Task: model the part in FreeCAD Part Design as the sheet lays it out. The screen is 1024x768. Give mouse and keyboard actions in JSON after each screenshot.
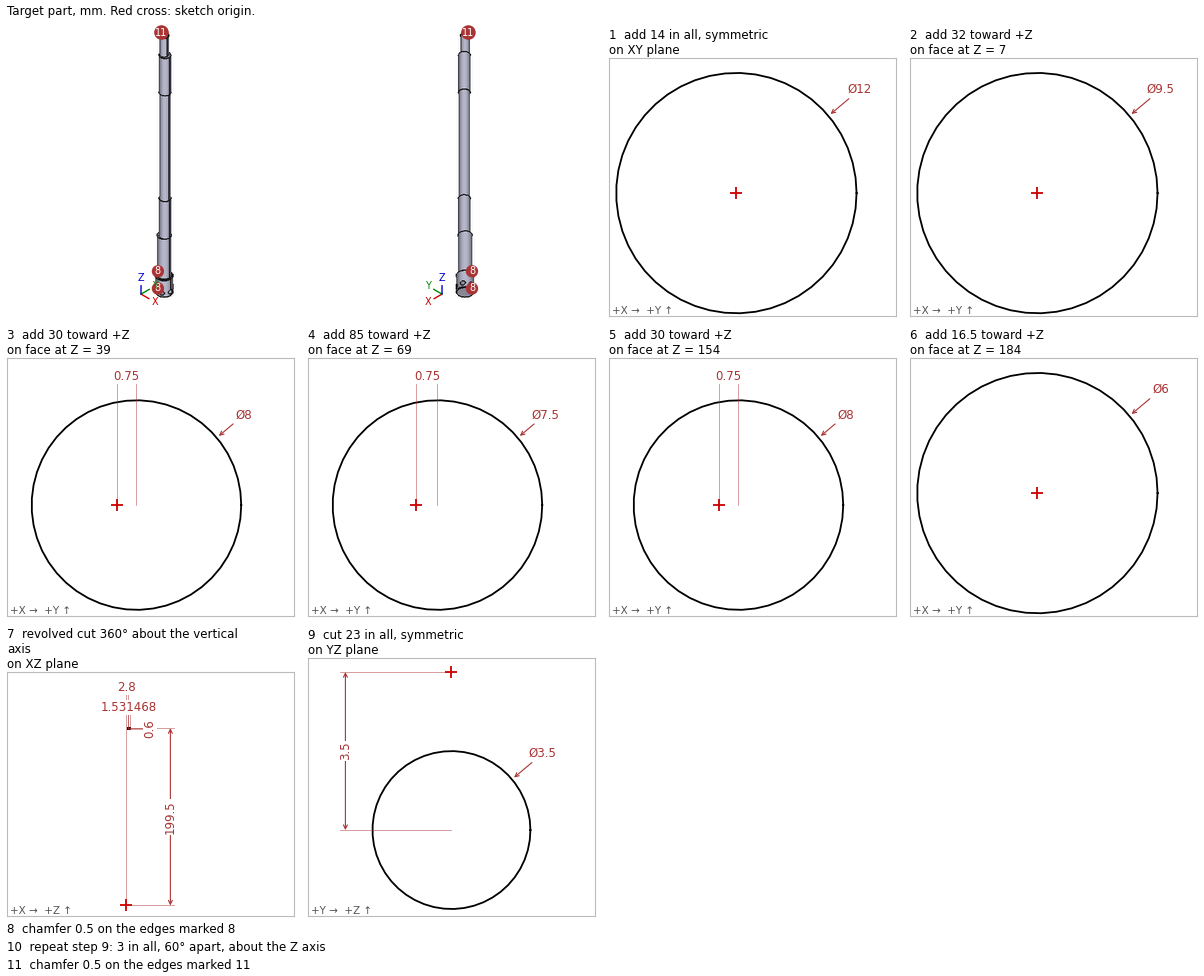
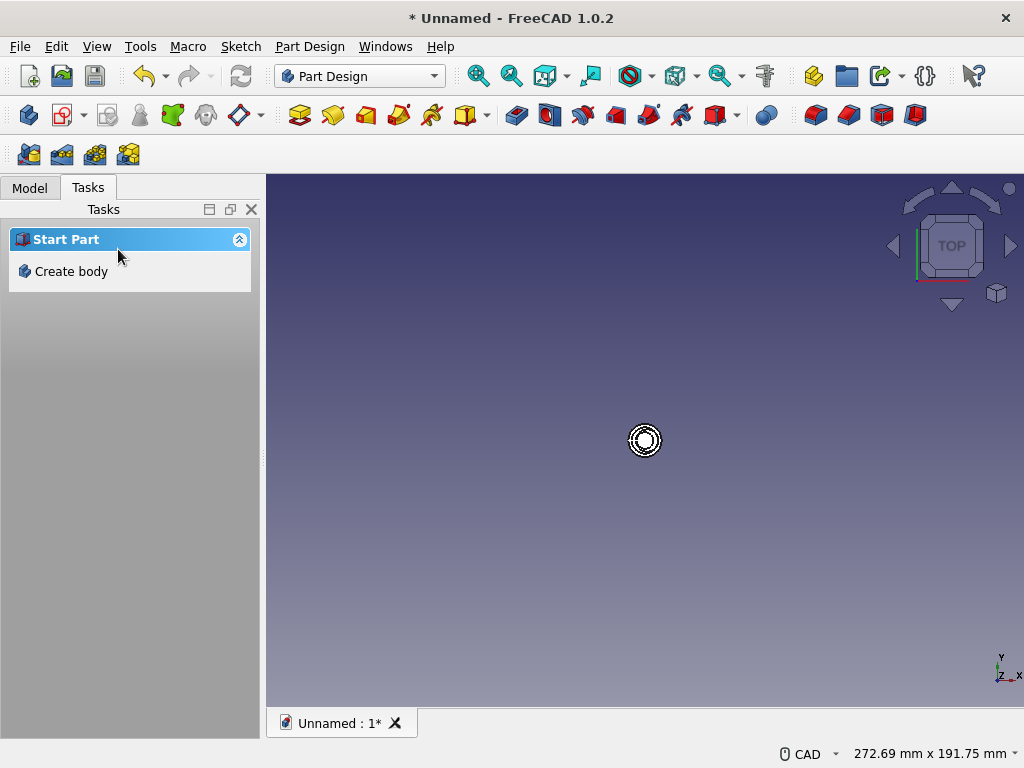
{"action": "key", "text": "v f"}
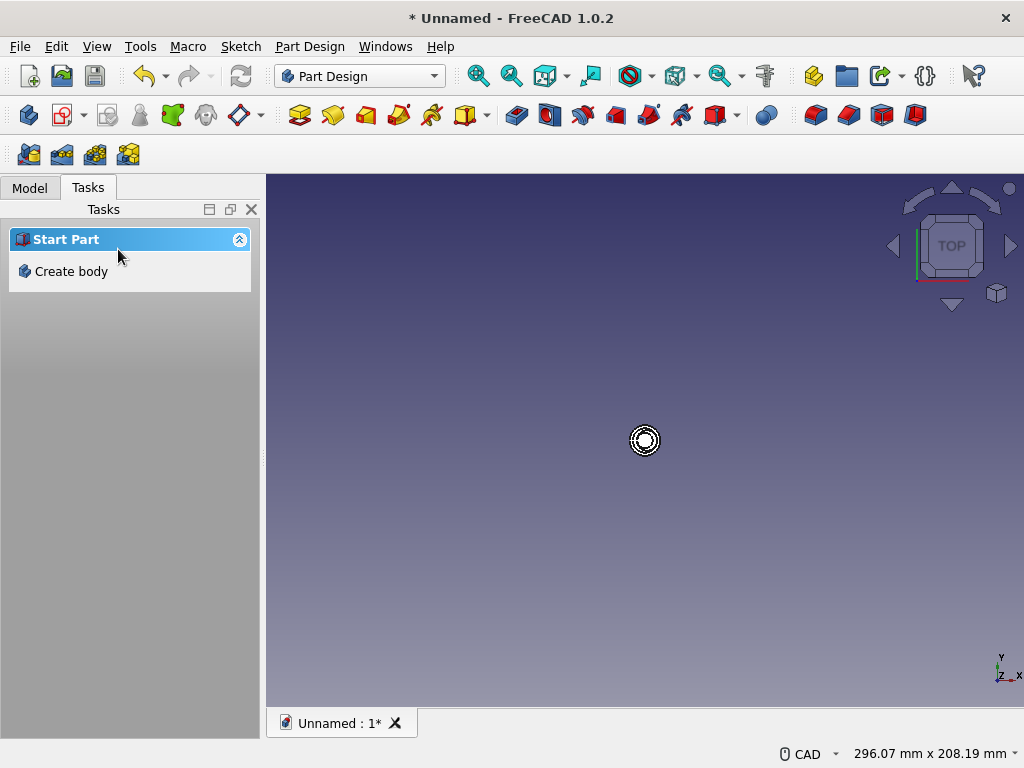
{"action": "left_click", "coordinate": [62, 116]}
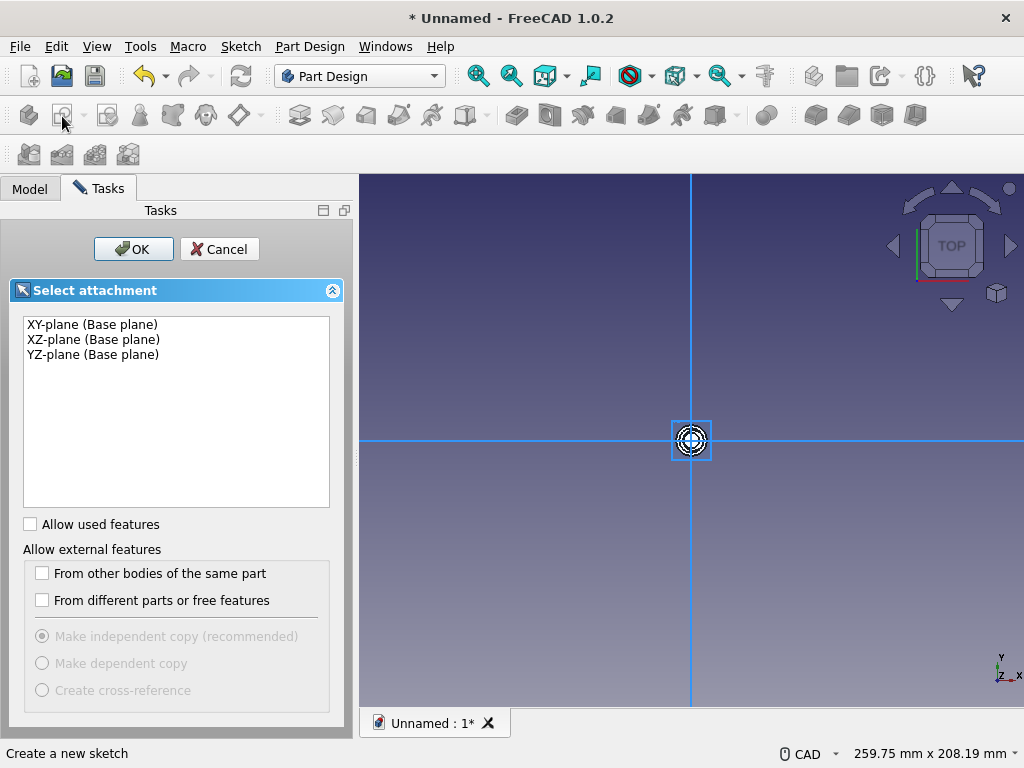
{"action": "left_click", "coordinate": [84, 340]}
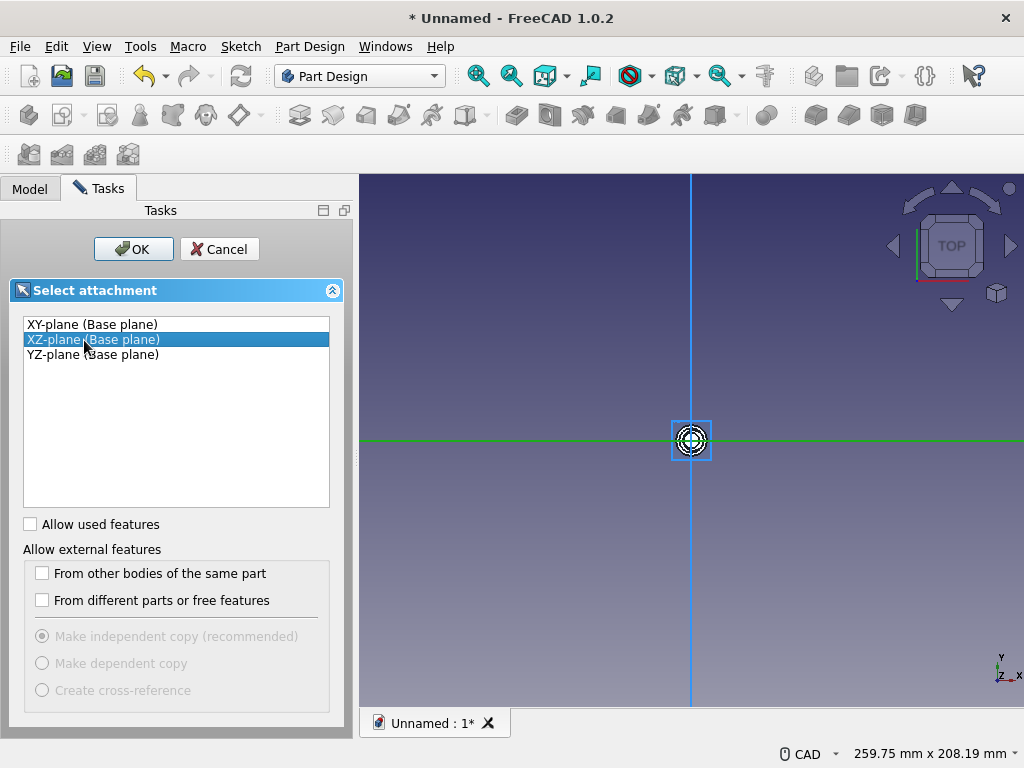
{"action": "left_click", "coordinate": [134, 249]}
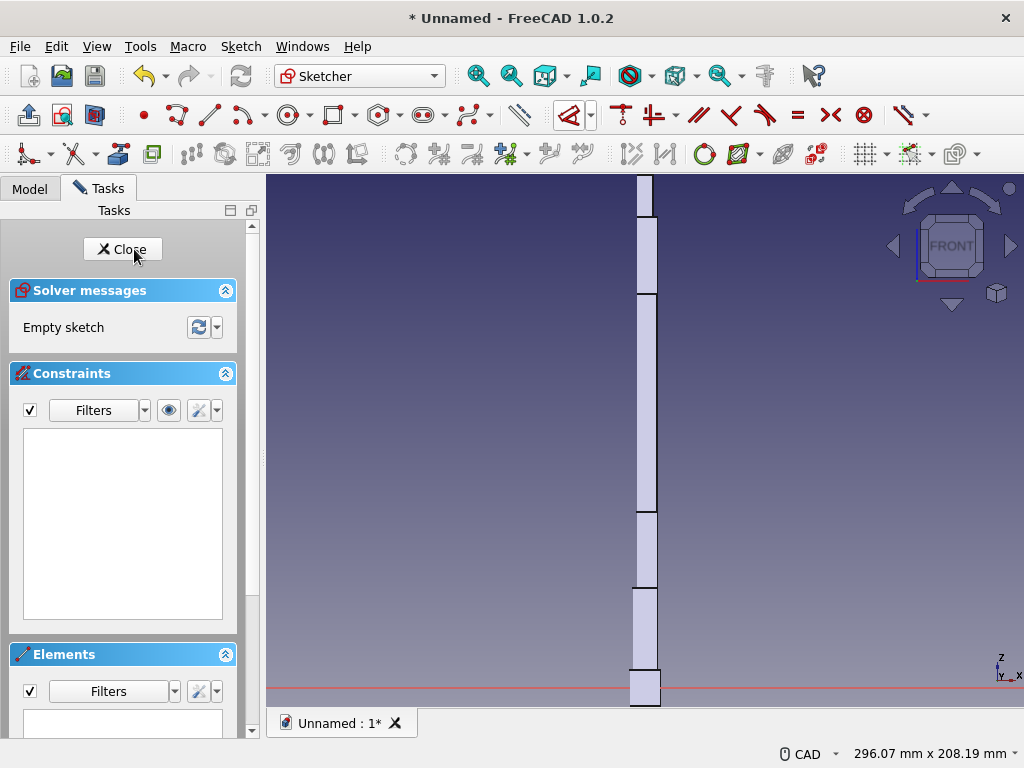
{"action": "left_click", "coordinate": [95, 116]}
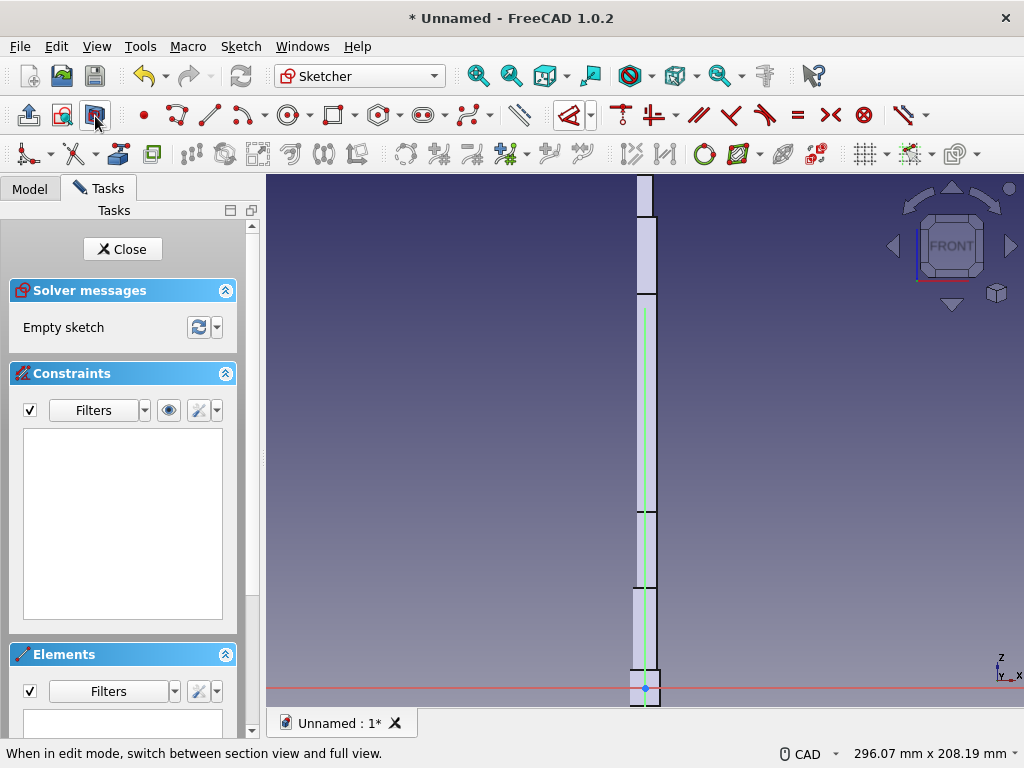
{"action": "scroll", "coordinate": [576, 440], "scroll_direction": "down", "scroll_amount": 5}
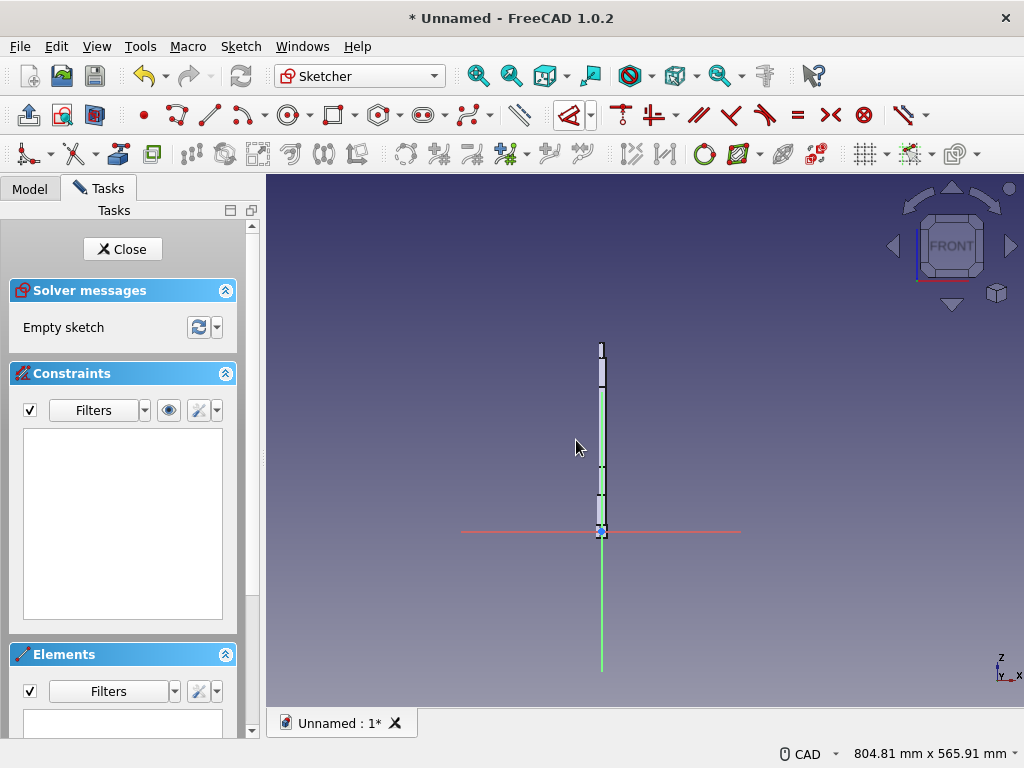
{"action": "scroll", "coordinate": [606, 339], "scroll_direction": "up", "scroll_amount": 15}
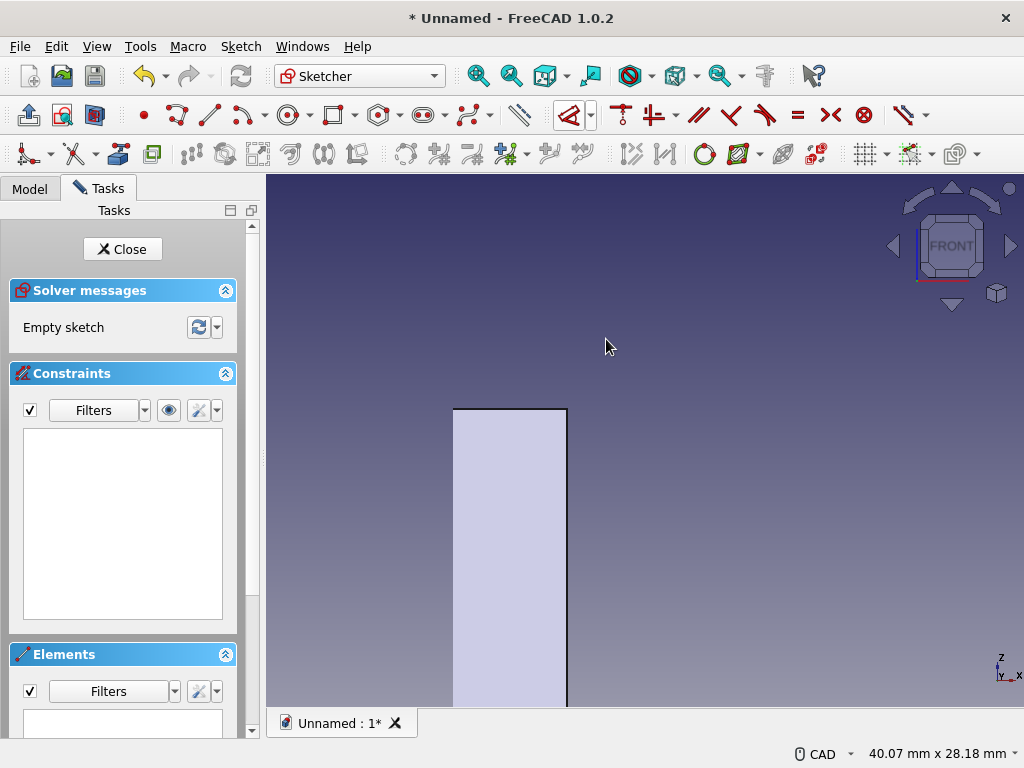
{"action": "scroll", "coordinate": [577, 433], "scroll_direction": "up", "scroll_amount": 13}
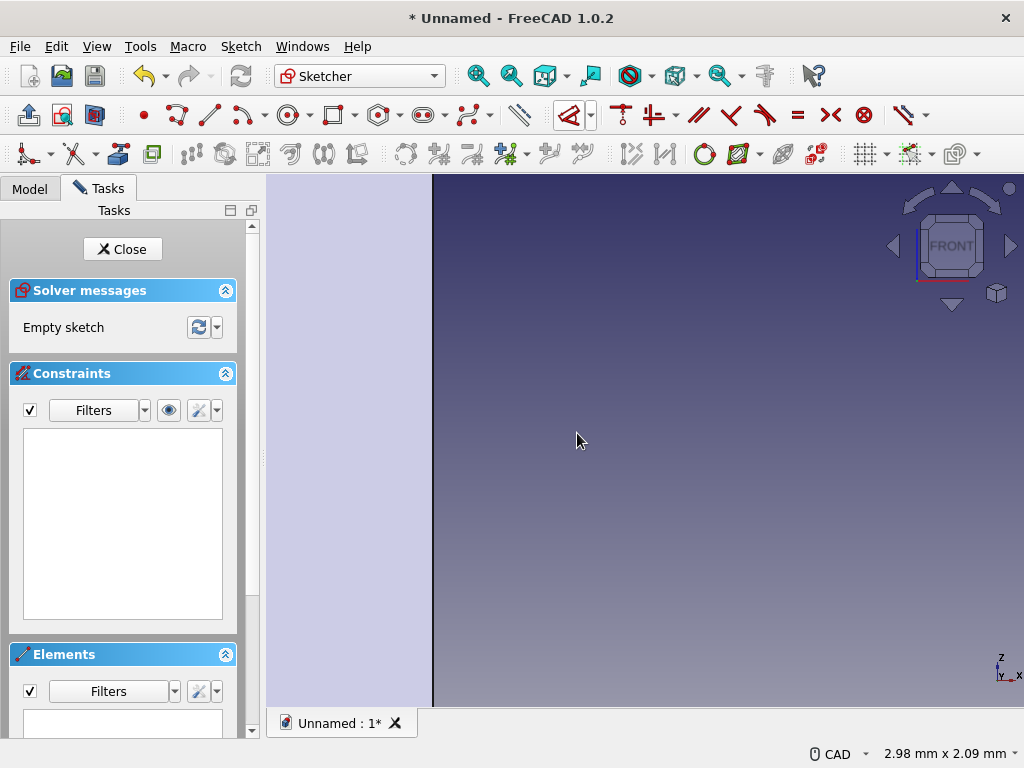
{"action": "key", "text": "g r"}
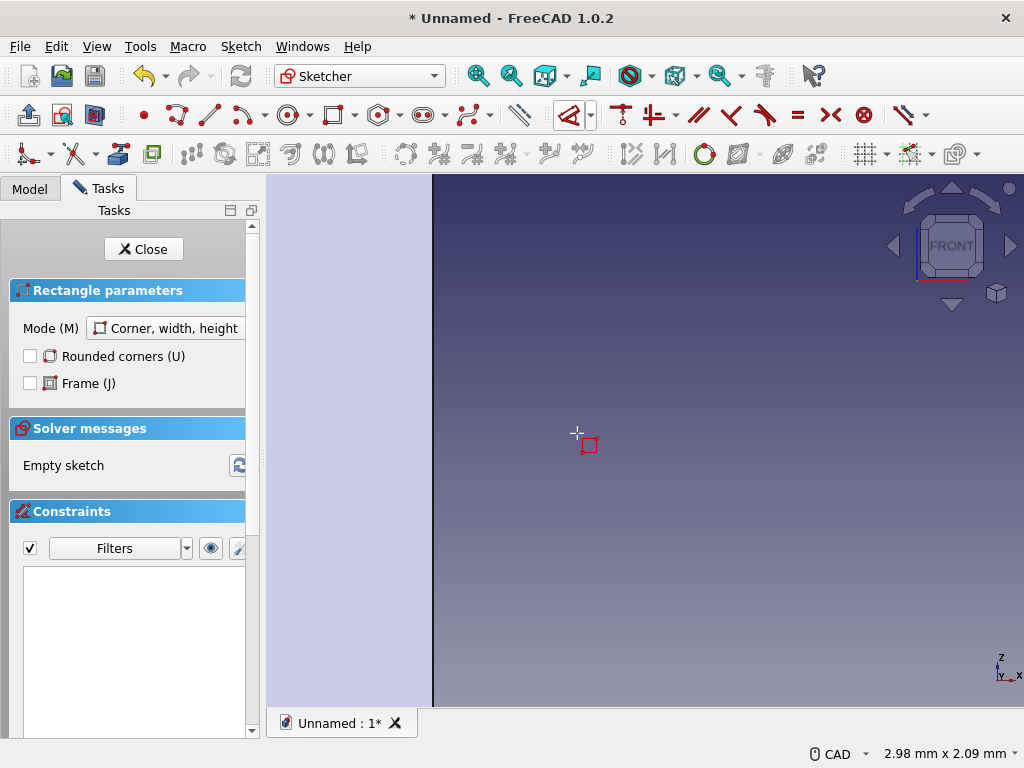
{"action": "left_click", "coordinate": [382, 360]}
{"action": "left_click", "coordinate": [772, 512]}
{"action": "key", "text": "Escape"}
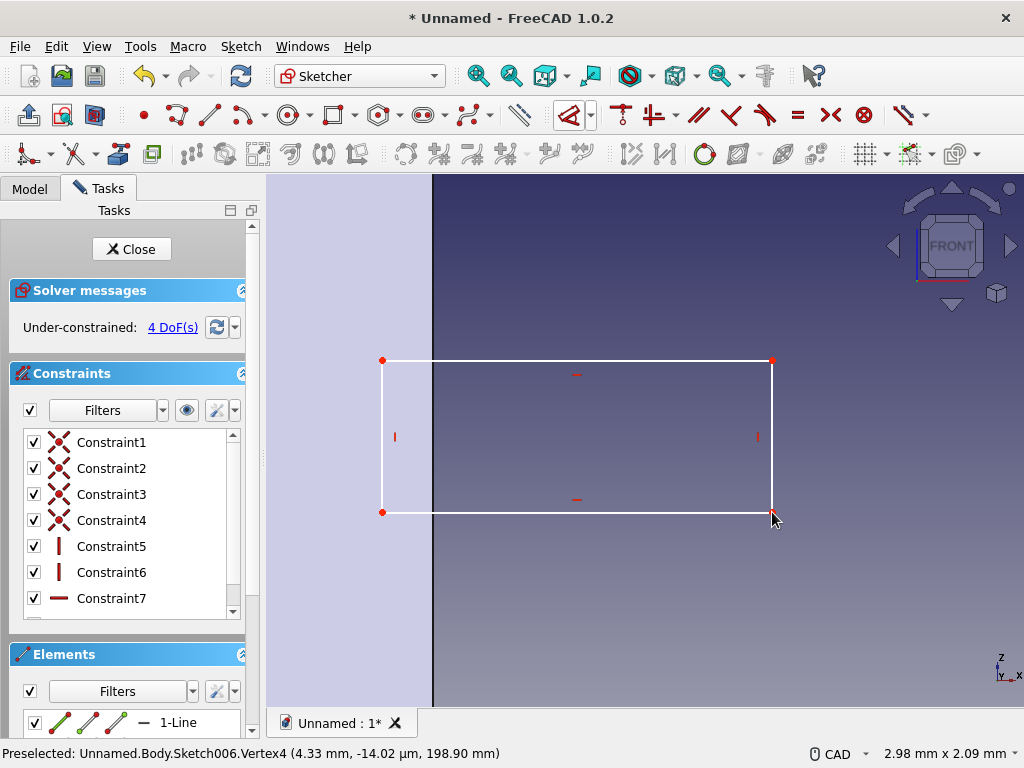
{"action": "left_click", "coordinate": [382, 407]}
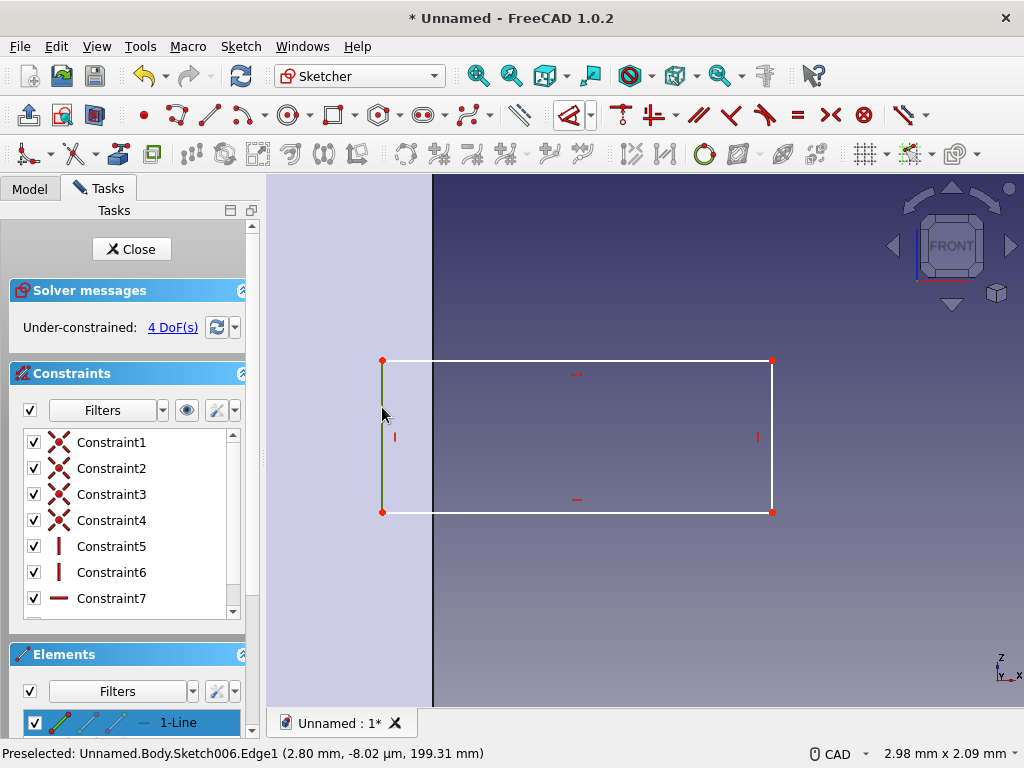
{"action": "key", "text": "i"}